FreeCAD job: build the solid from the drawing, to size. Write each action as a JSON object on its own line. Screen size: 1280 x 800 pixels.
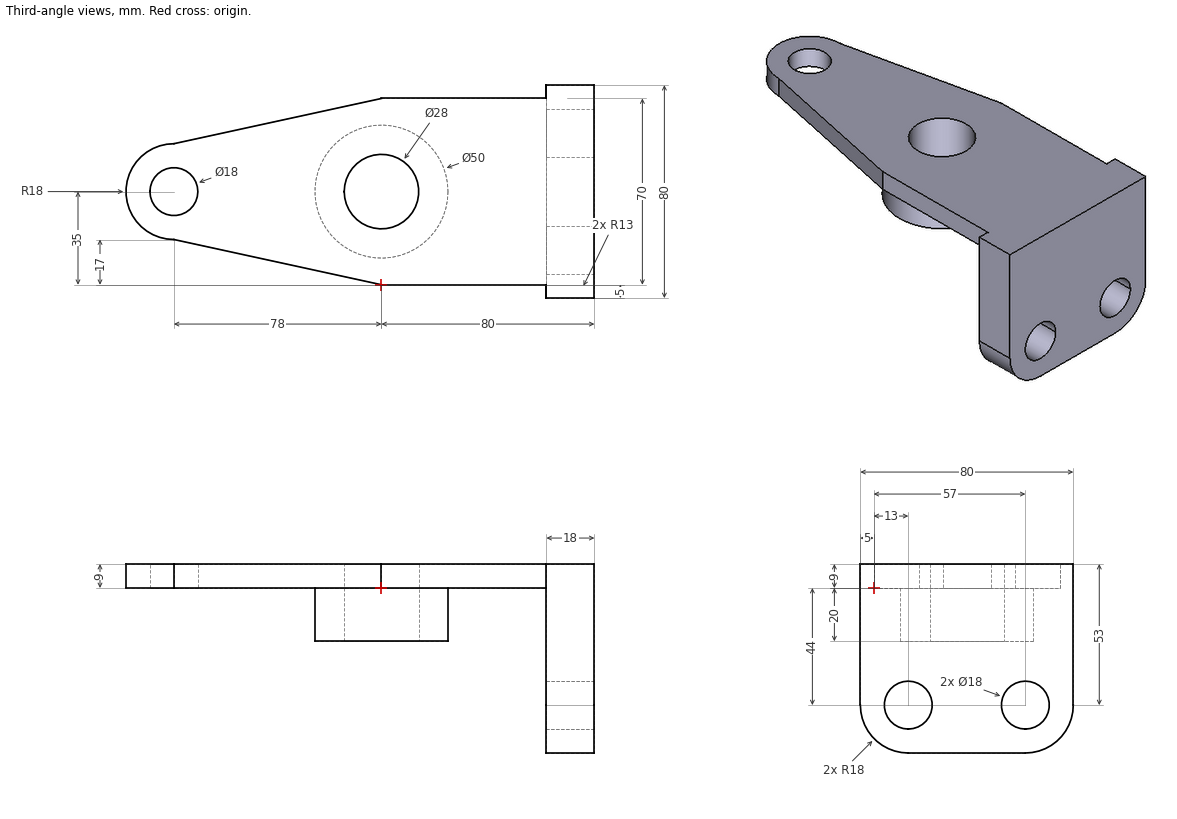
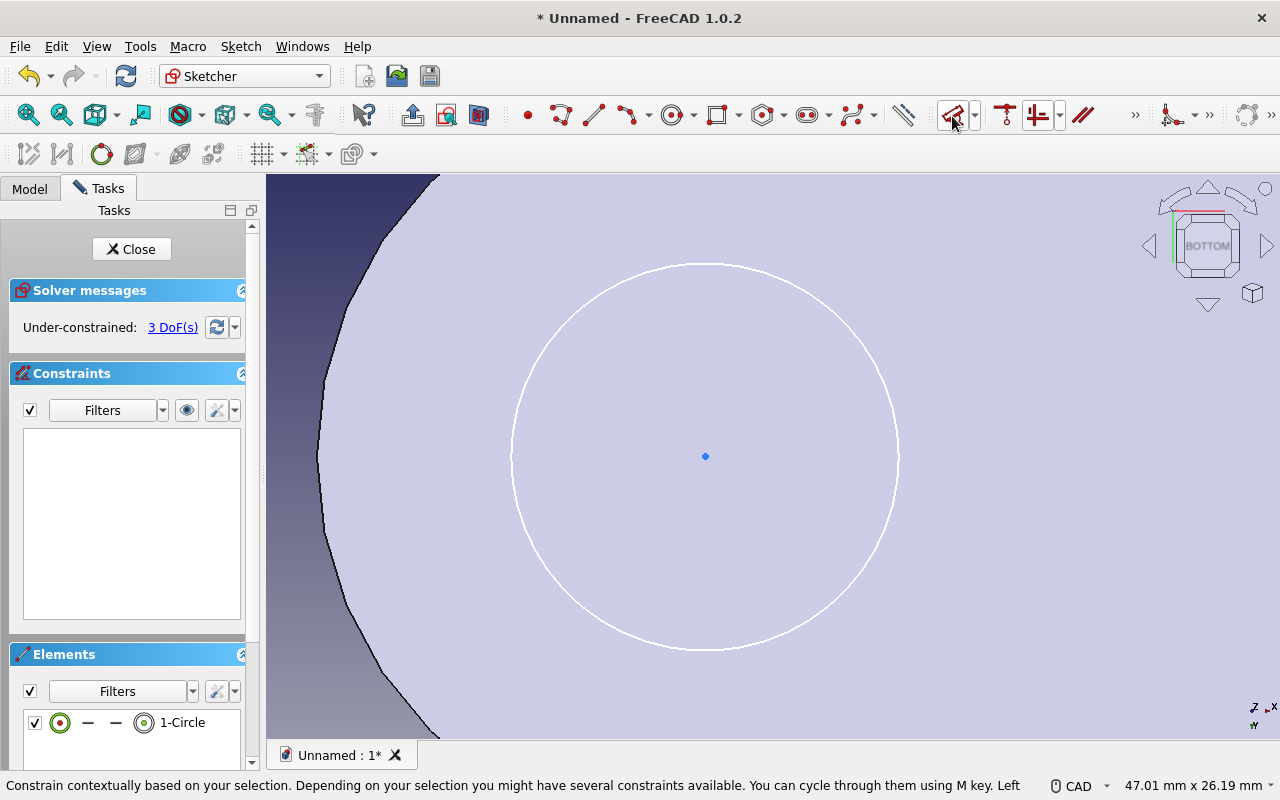
{"action": "left_click", "coordinate": [842, 320]}
{"action": "left_click", "coordinate": [865, 297]}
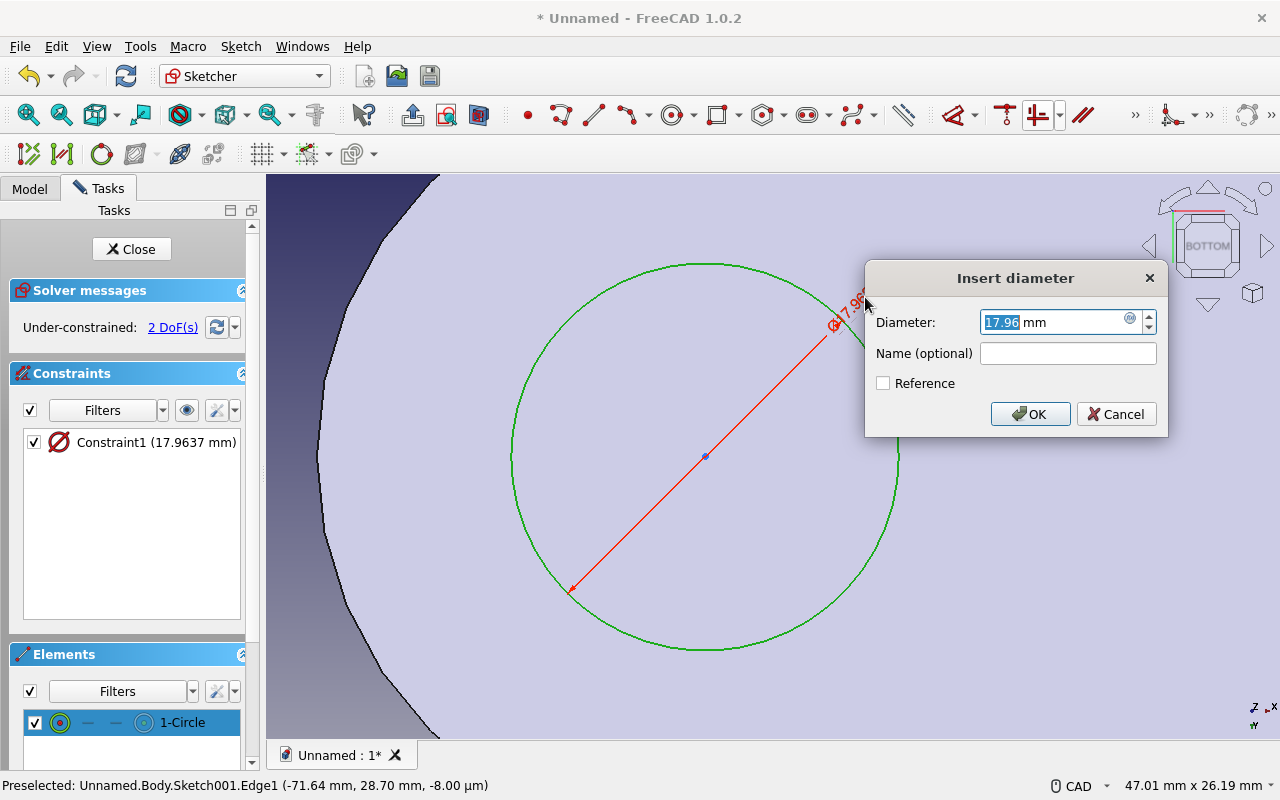
{"action": "type", "text": "18"}
{"action": "key", "text": "Return"}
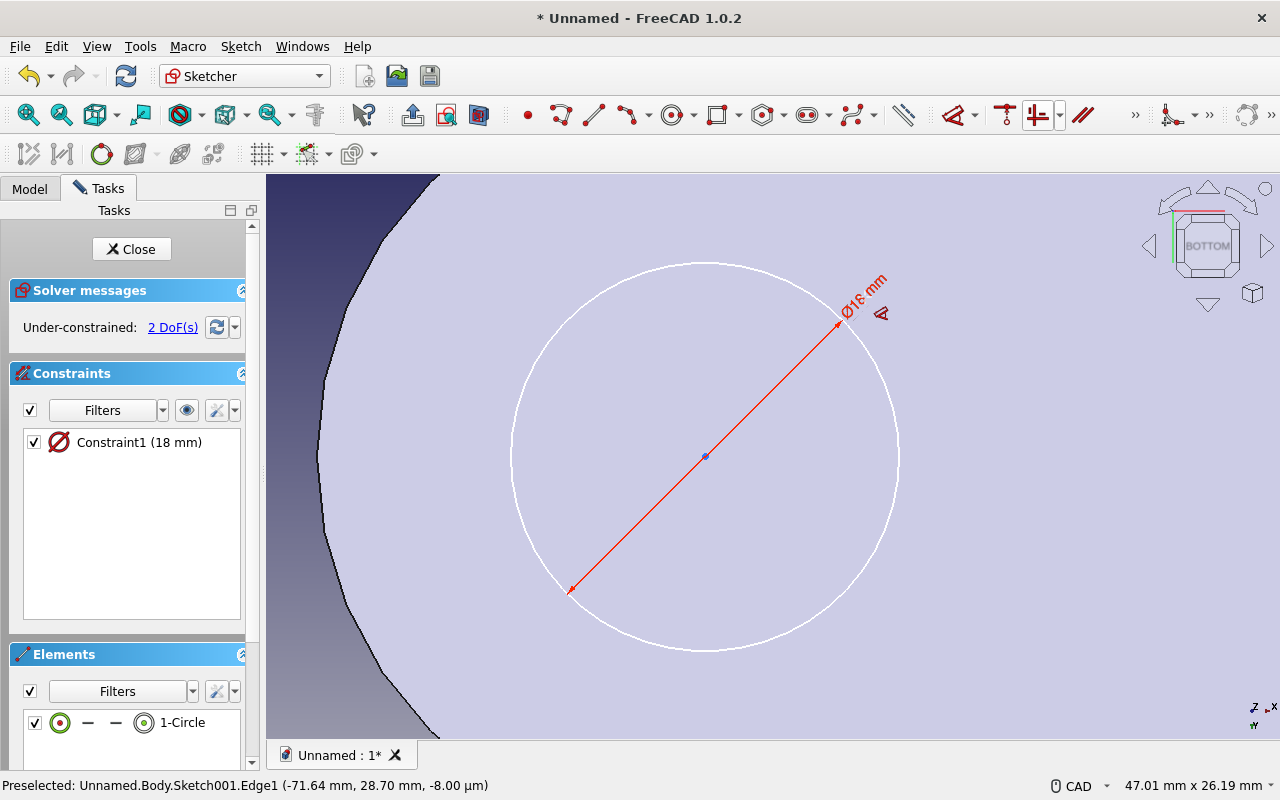
{"action": "left_click", "coordinate": [705, 457]}
{"action": "left_click", "coordinate": [910, 491]}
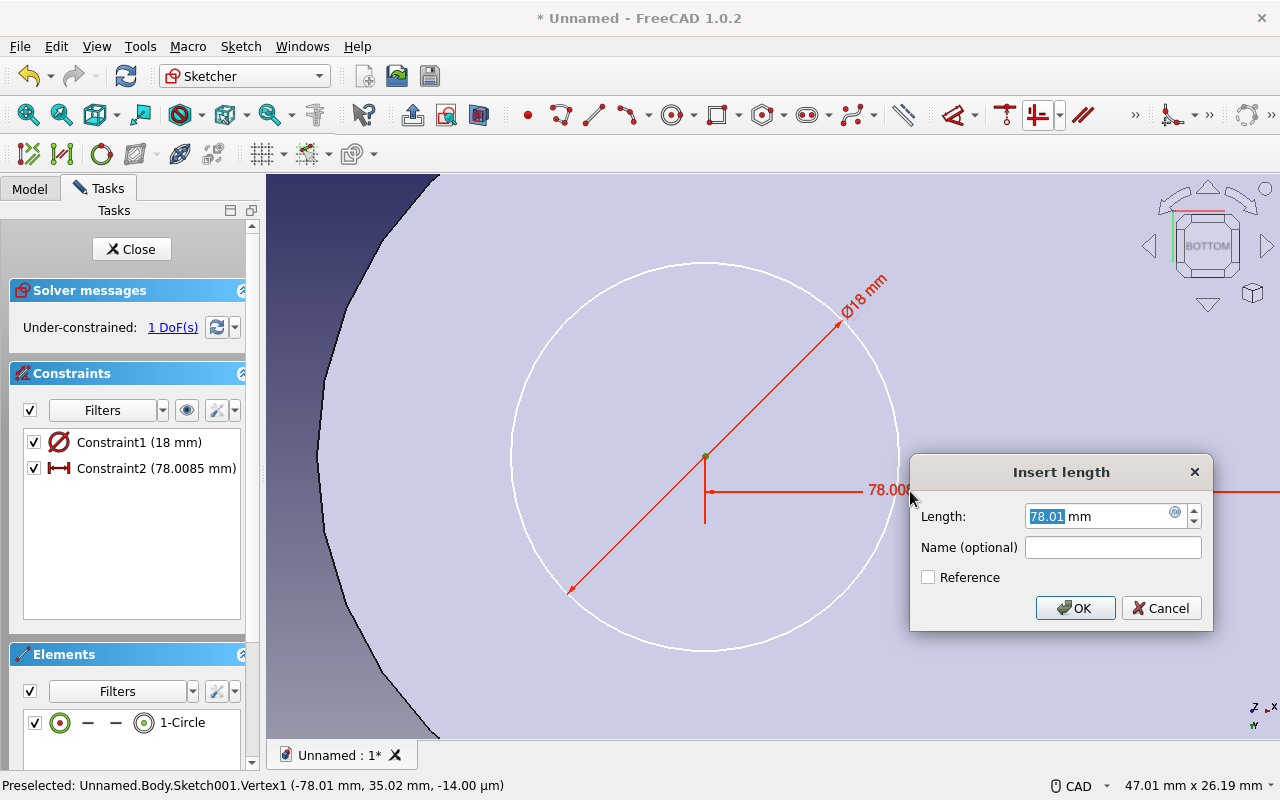
{"action": "type", "text": "78"}
{"action": "key", "text": "Return"}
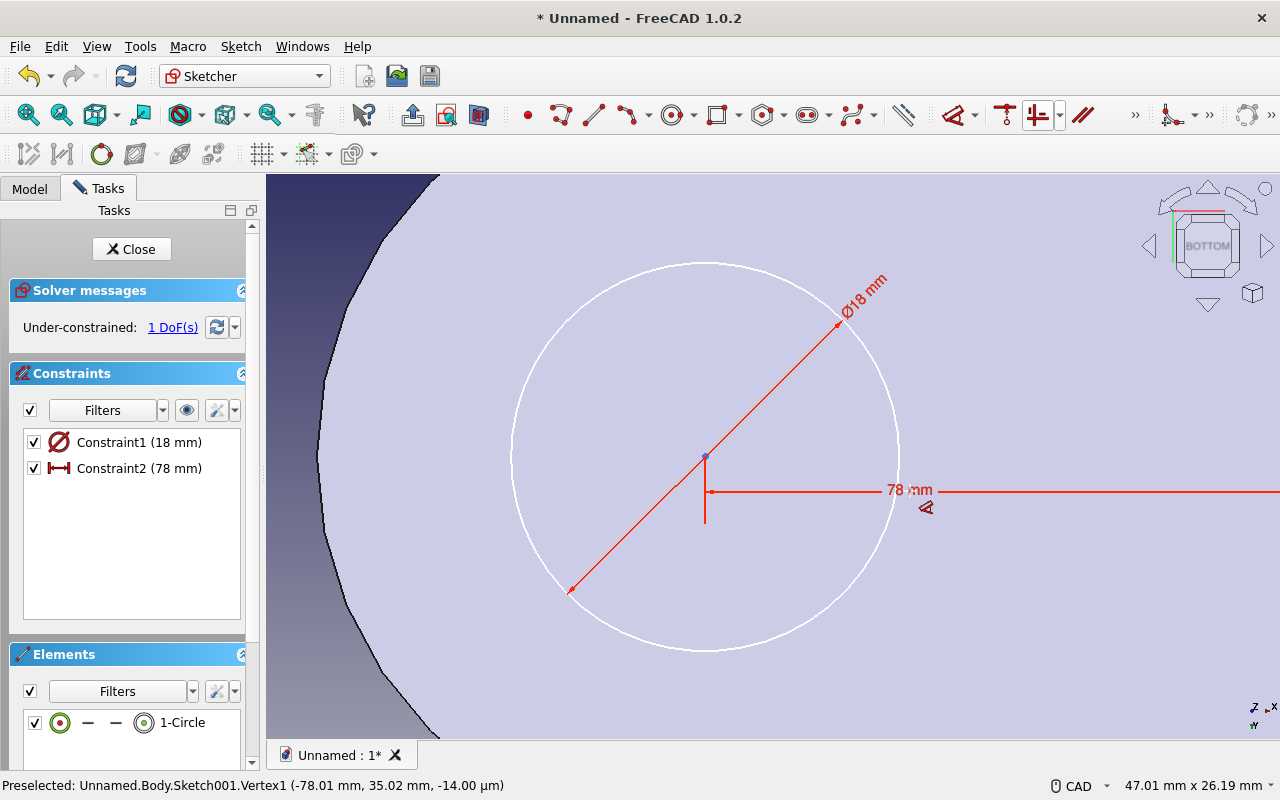
{"action": "left_click", "coordinate": [705, 457]}
{"action": "left_click", "coordinate": [671, 329]}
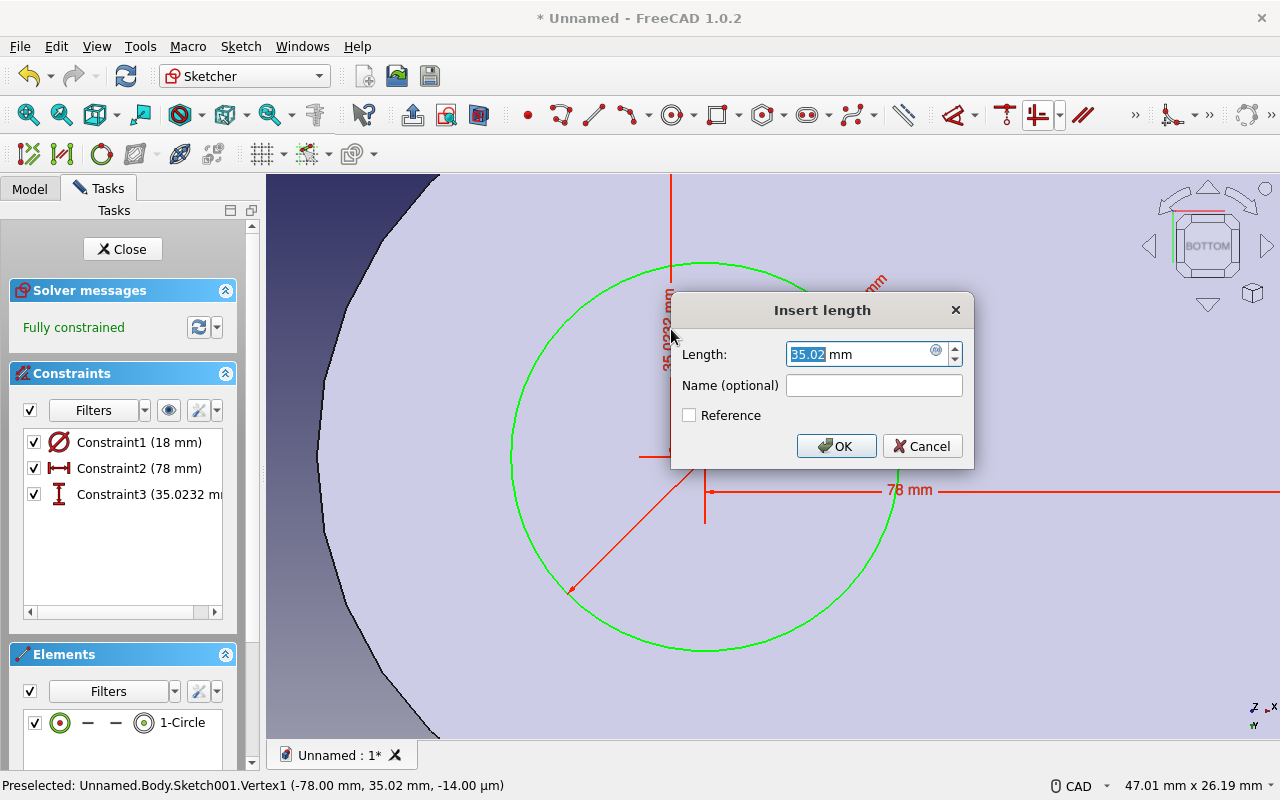
{"action": "type", "text": "35"}
{"action": "key", "text": "Return"}
{"action": "key", "text": "Escape"}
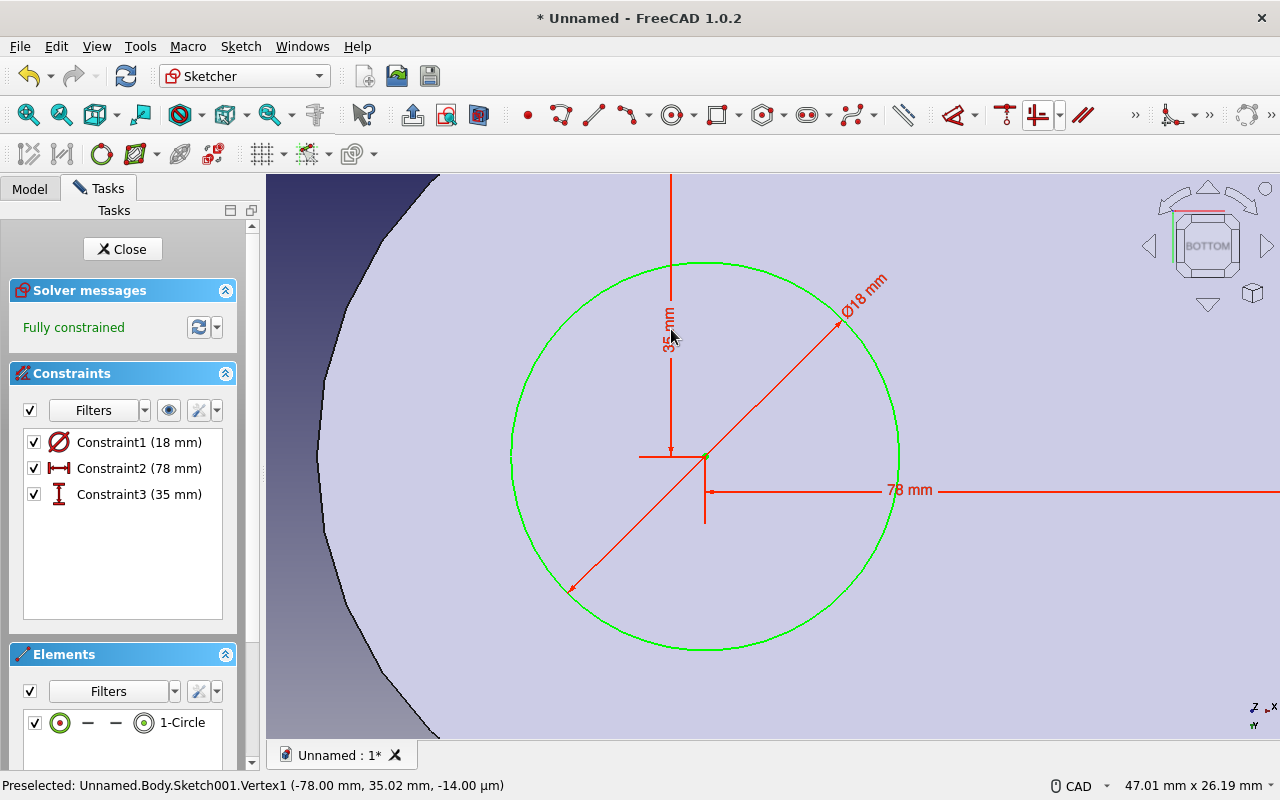
{"action": "left_click", "coordinate": [123, 249]}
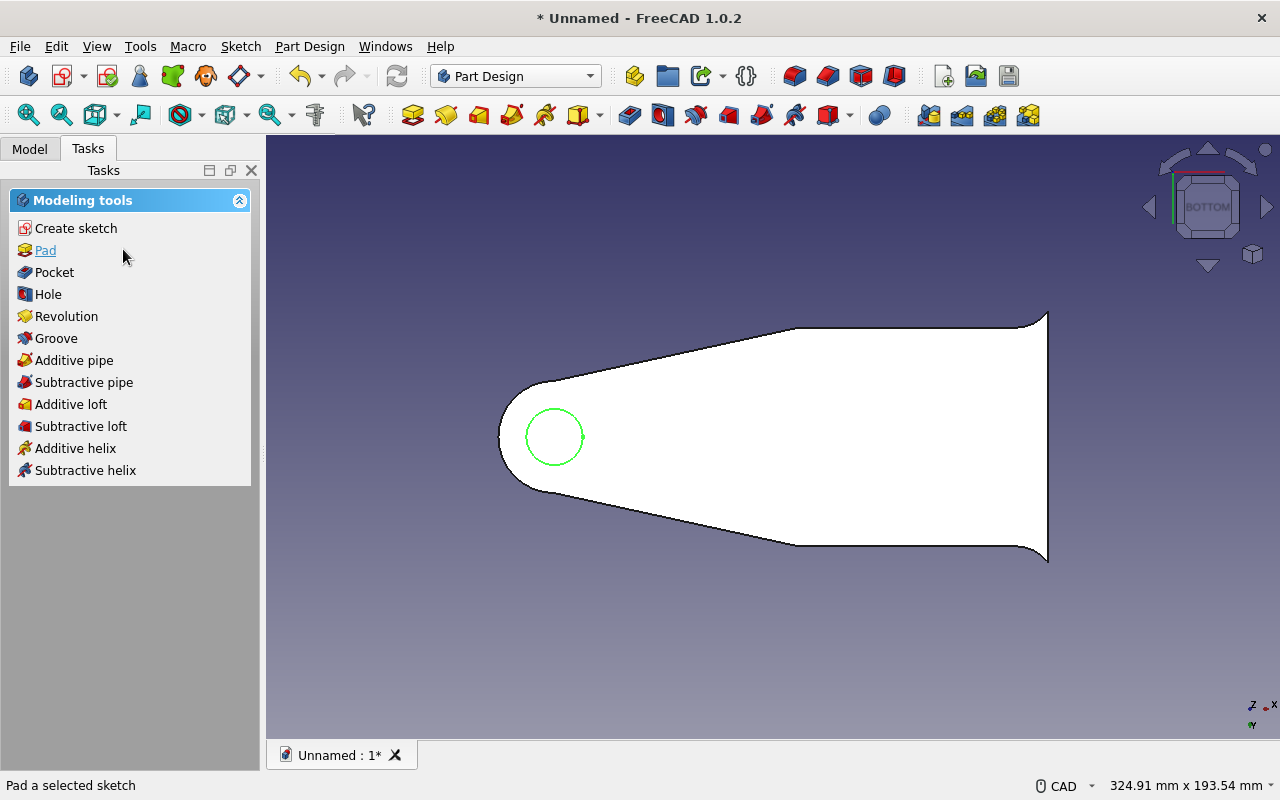
{"action": "left_click", "coordinate": [630, 116]}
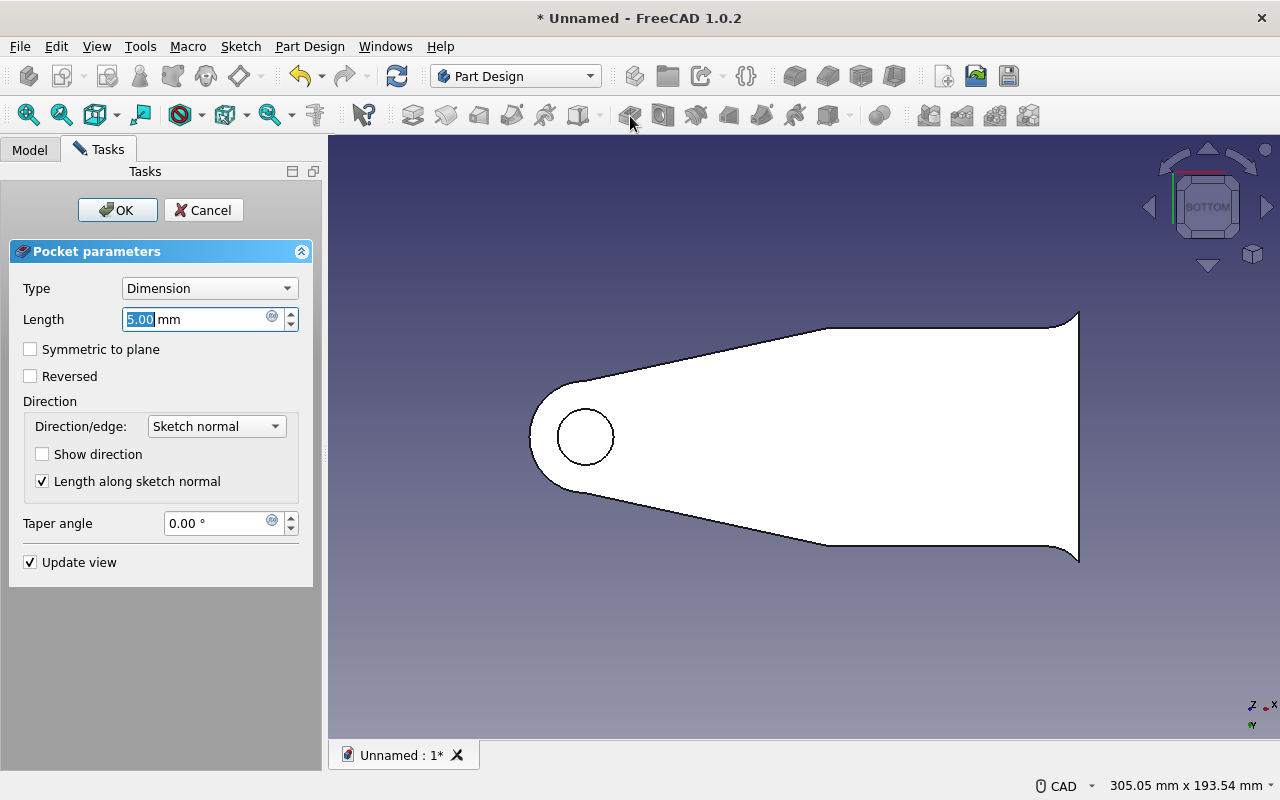
{"action": "type", "text": "9"}
{"action": "key", "text": "Tab"}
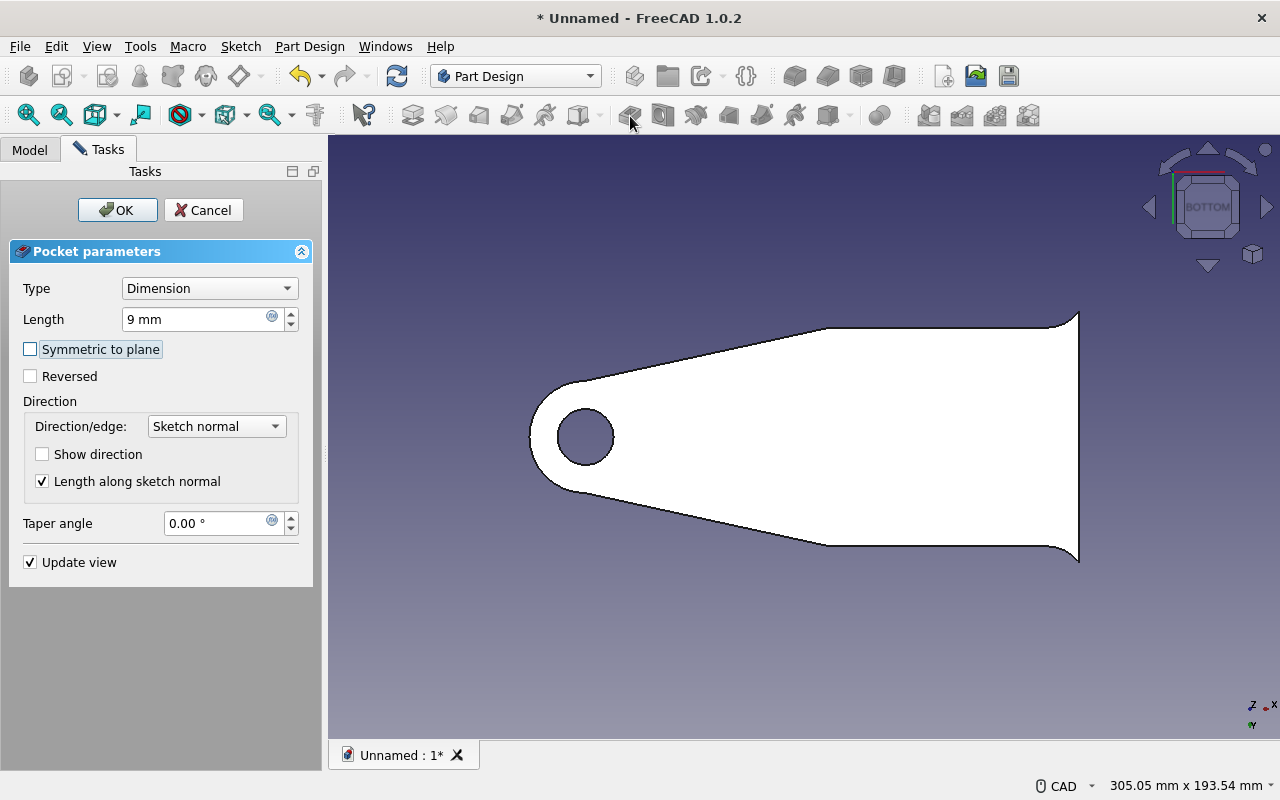
{"action": "left_click", "coordinate": [118, 210]}